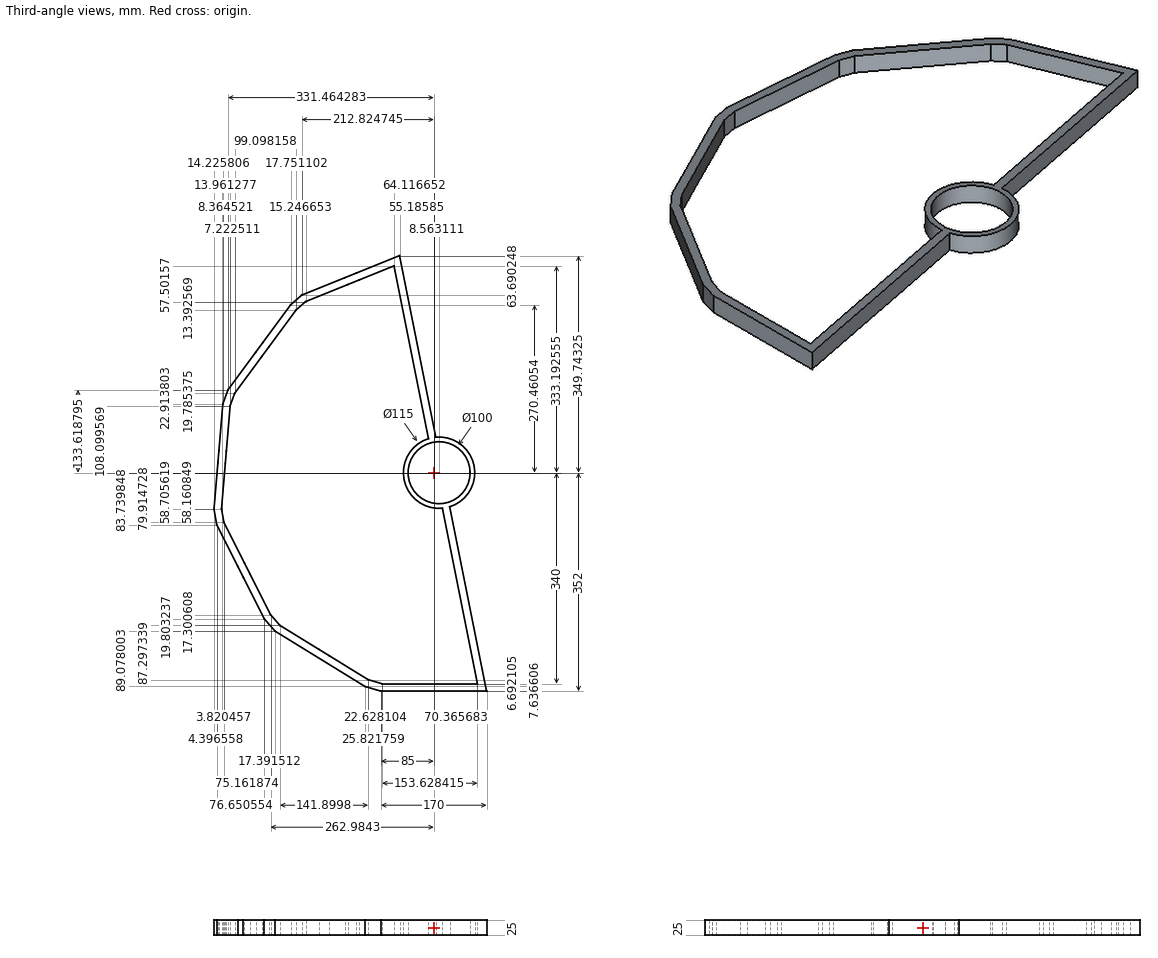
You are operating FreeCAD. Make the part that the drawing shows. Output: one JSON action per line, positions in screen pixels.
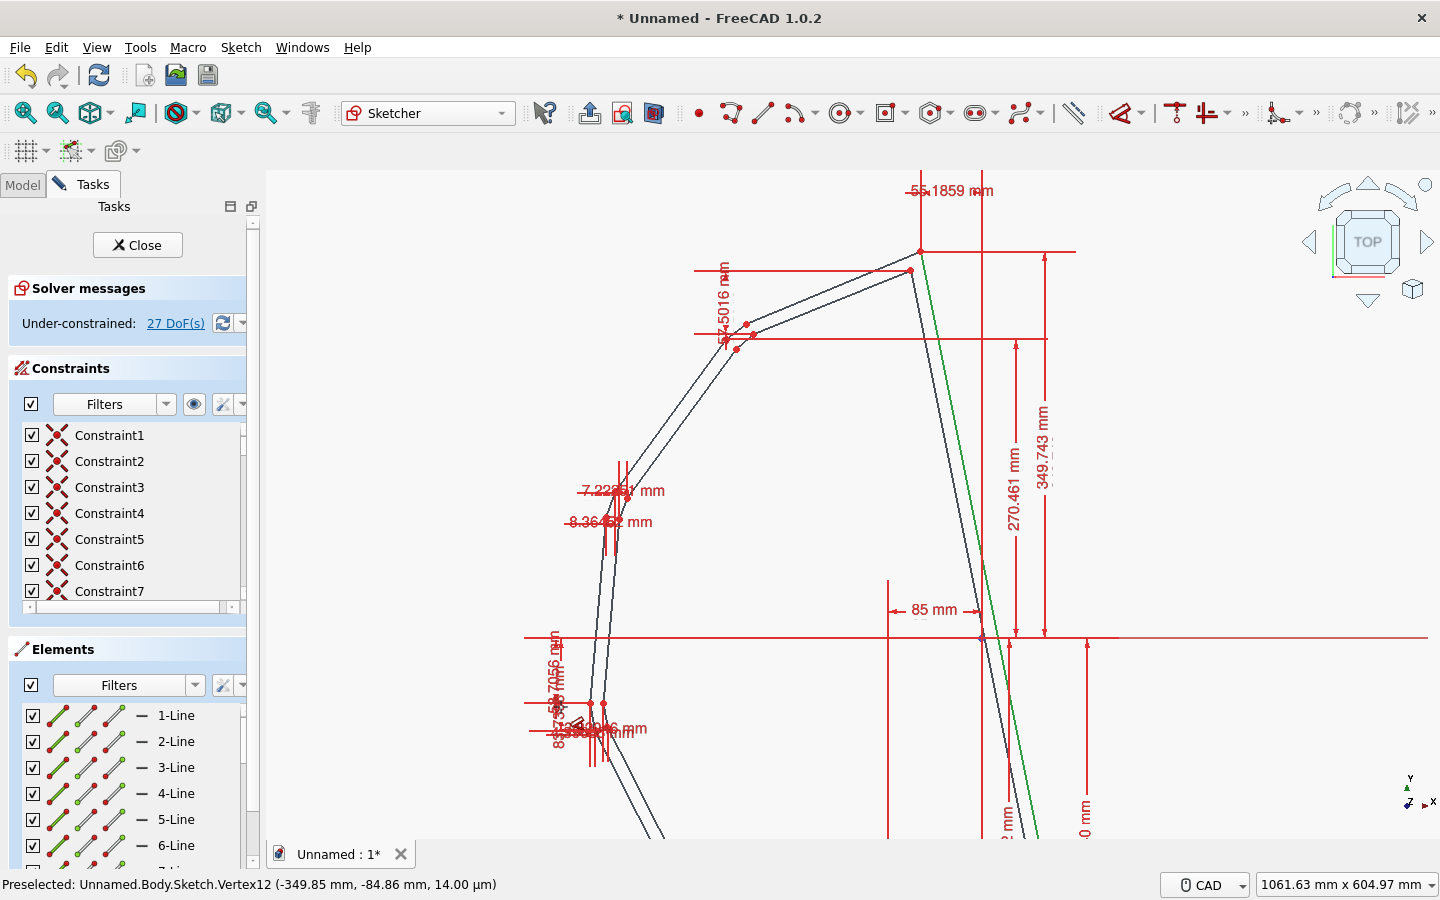
{"action": "left_click", "coordinate": [911, 271]}
{"action": "left_click", "coordinate": [946, 237]}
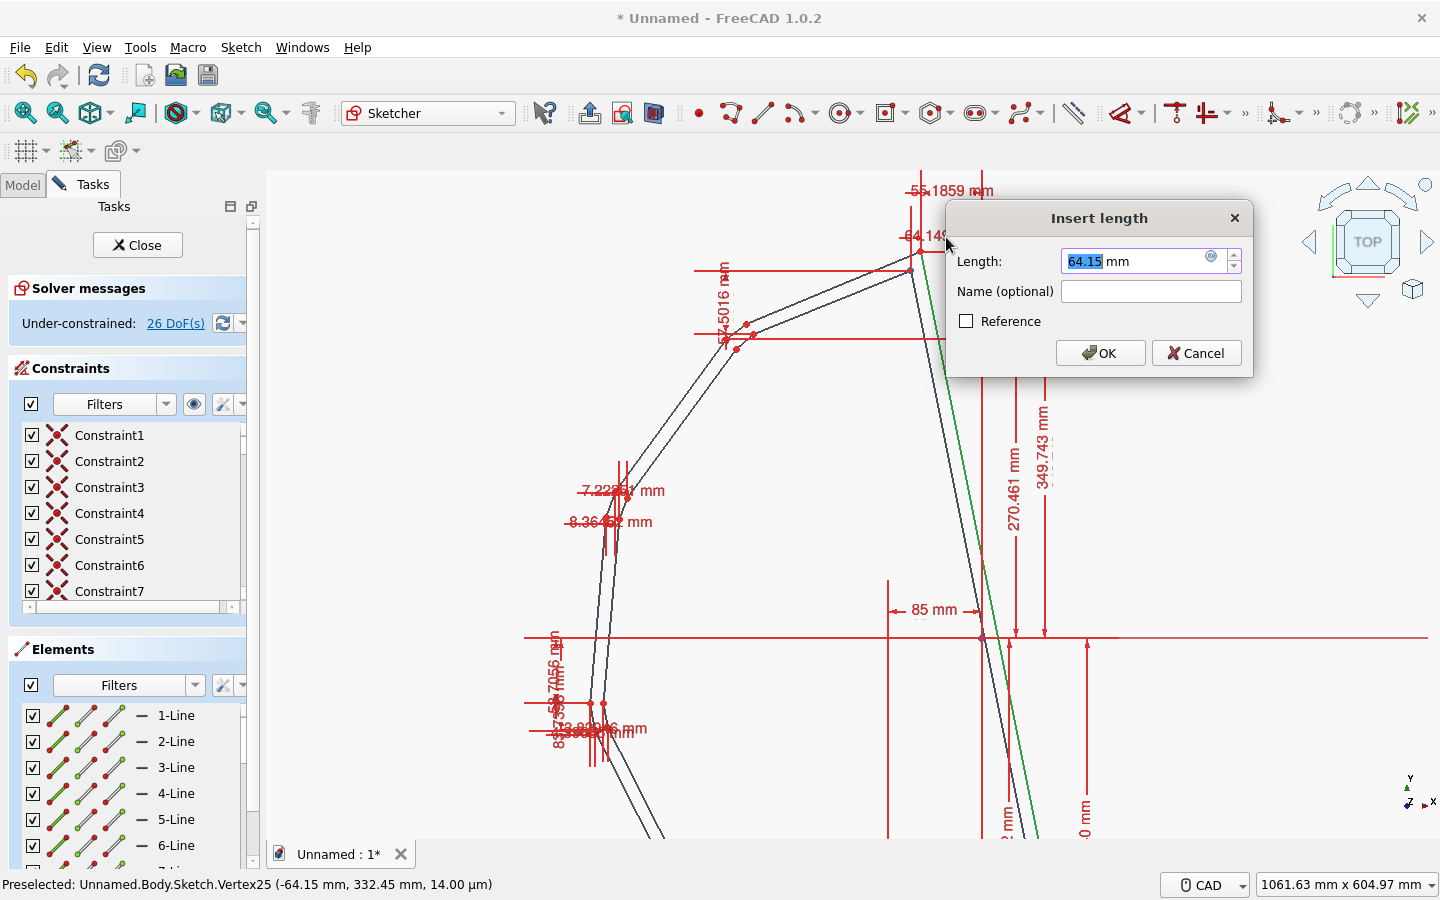
{"action": "type", "text": "64.116652"}
{"action": "key", "text": "Return"}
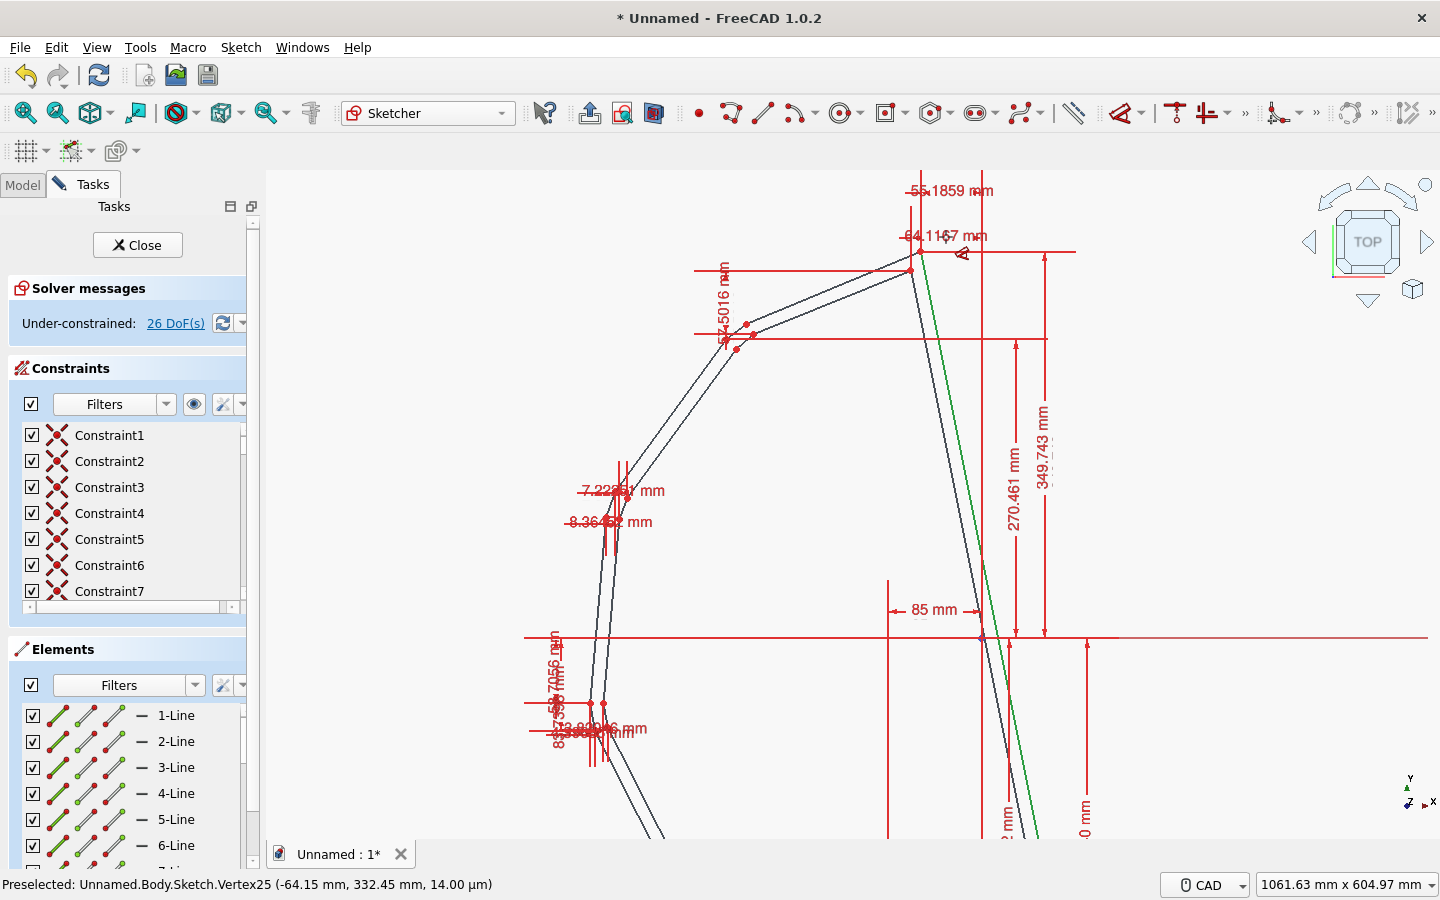
{"action": "scroll", "coordinate": [725, 340], "scroll_direction": "down", "scroll_amount": 3}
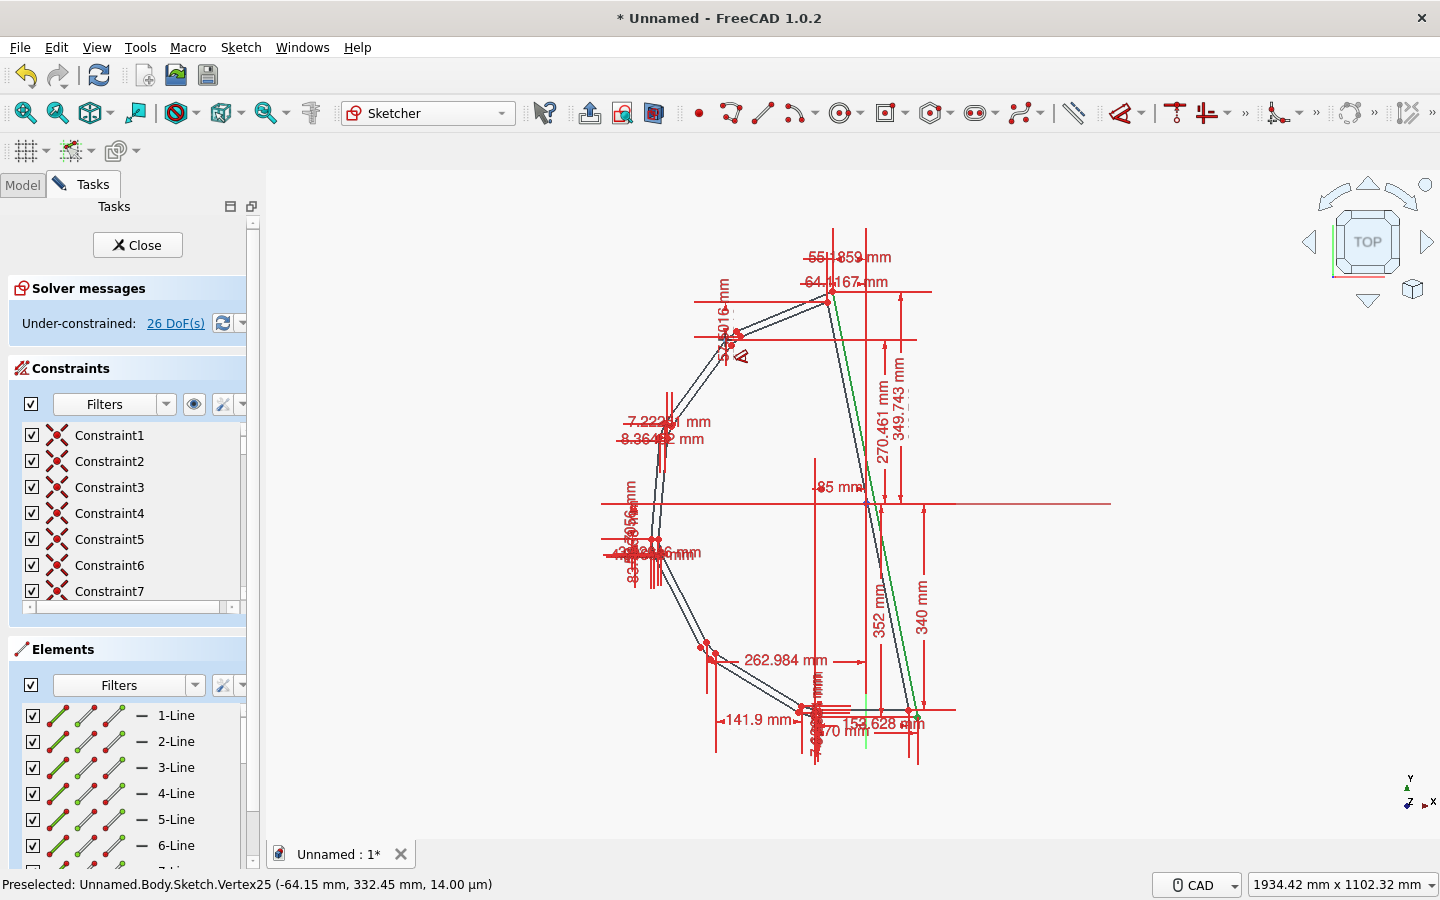
{"action": "left_click", "coordinate": [909, 710]}
{"action": "left_click", "coordinate": [888, 768]}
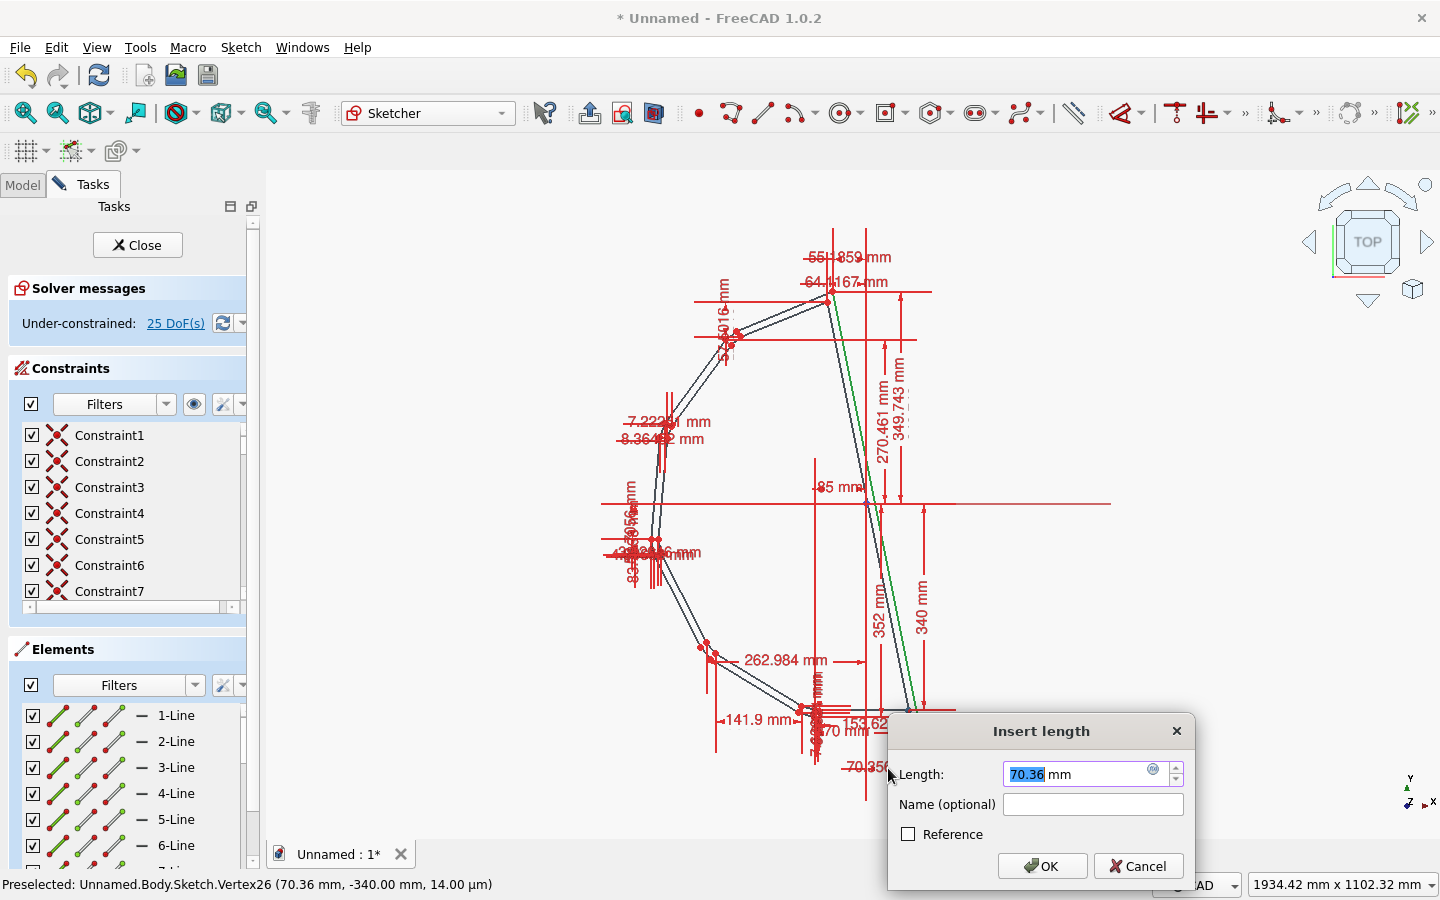
{"action": "type", "text": "70.365683"}
{"action": "key", "text": "Return"}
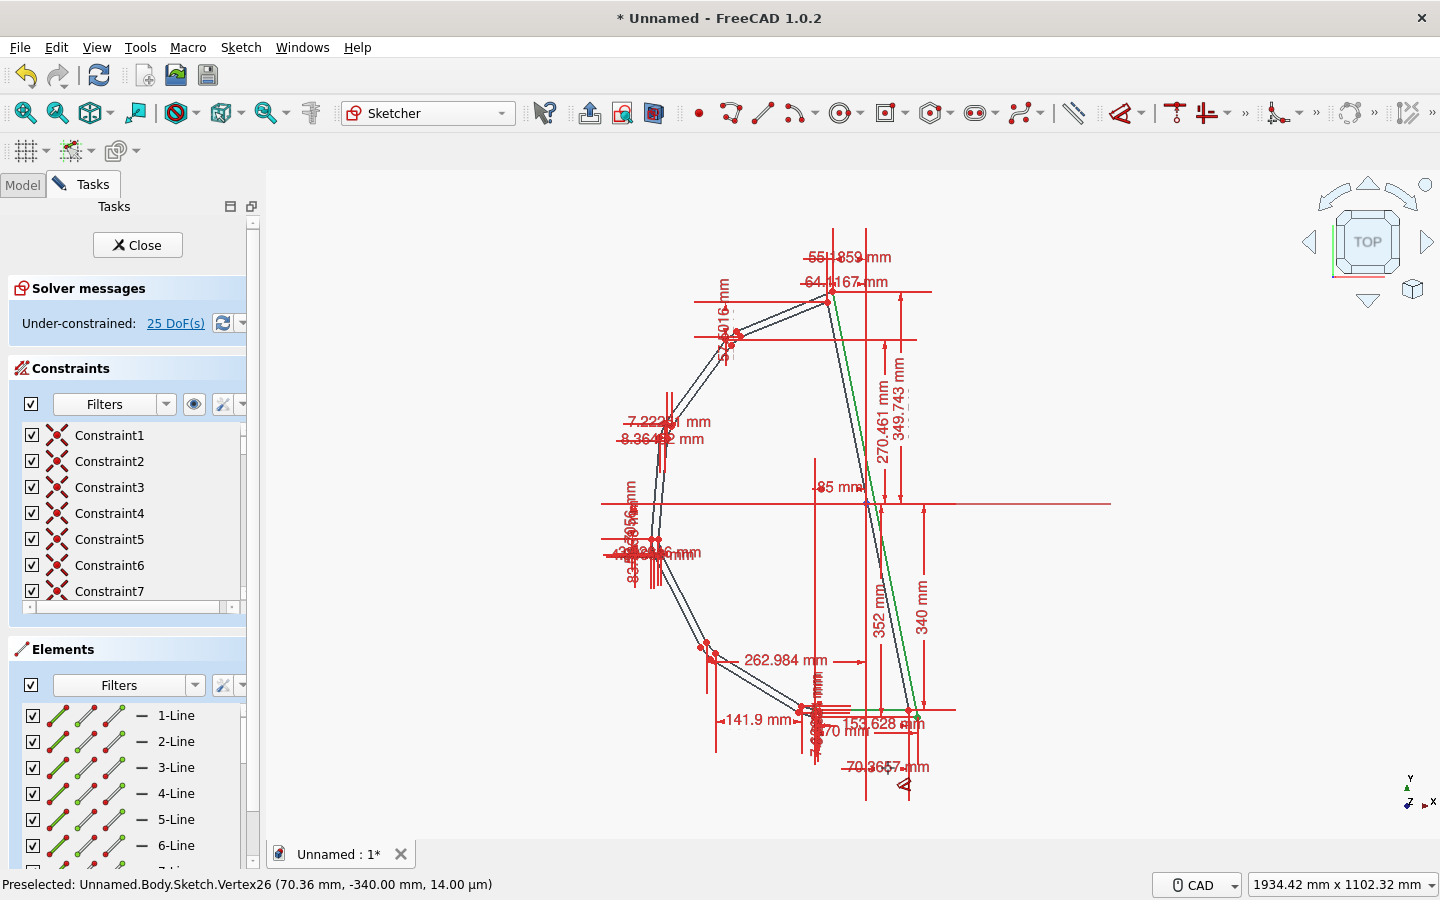
{"action": "scroll", "coordinate": [661, 553], "scroll_direction": "up", "scroll_amount": 3}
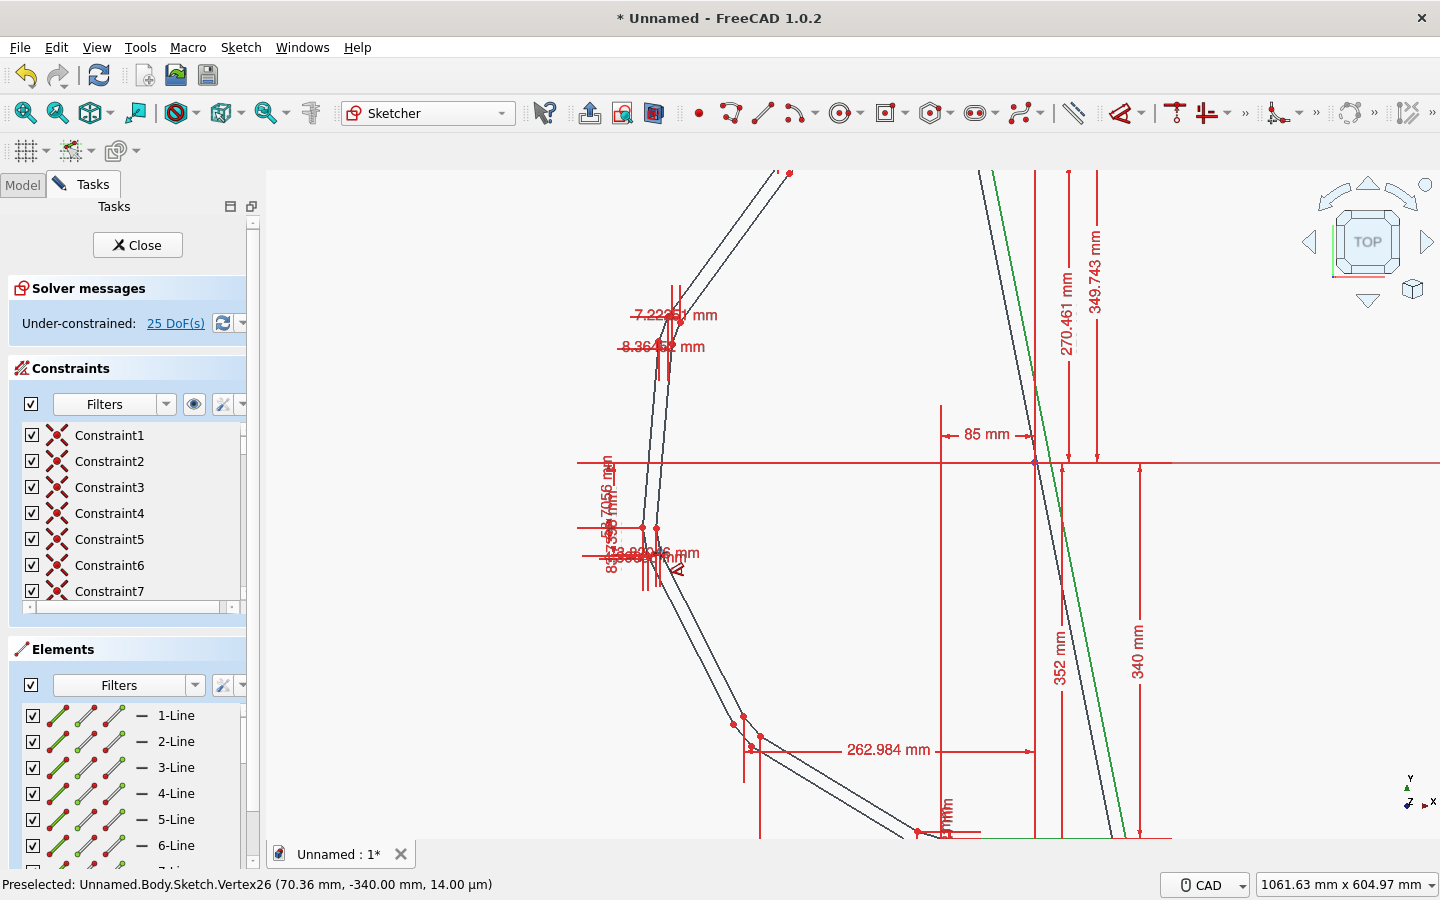
{"action": "left_click", "coordinate": [660, 552]}
{"action": "left_click", "coordinate": [1069, 476]}